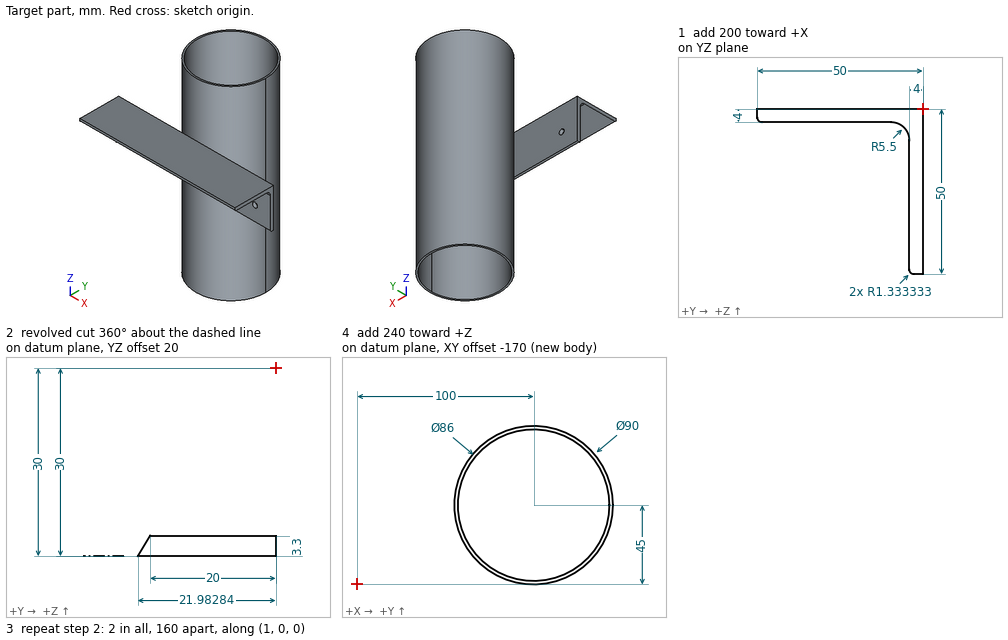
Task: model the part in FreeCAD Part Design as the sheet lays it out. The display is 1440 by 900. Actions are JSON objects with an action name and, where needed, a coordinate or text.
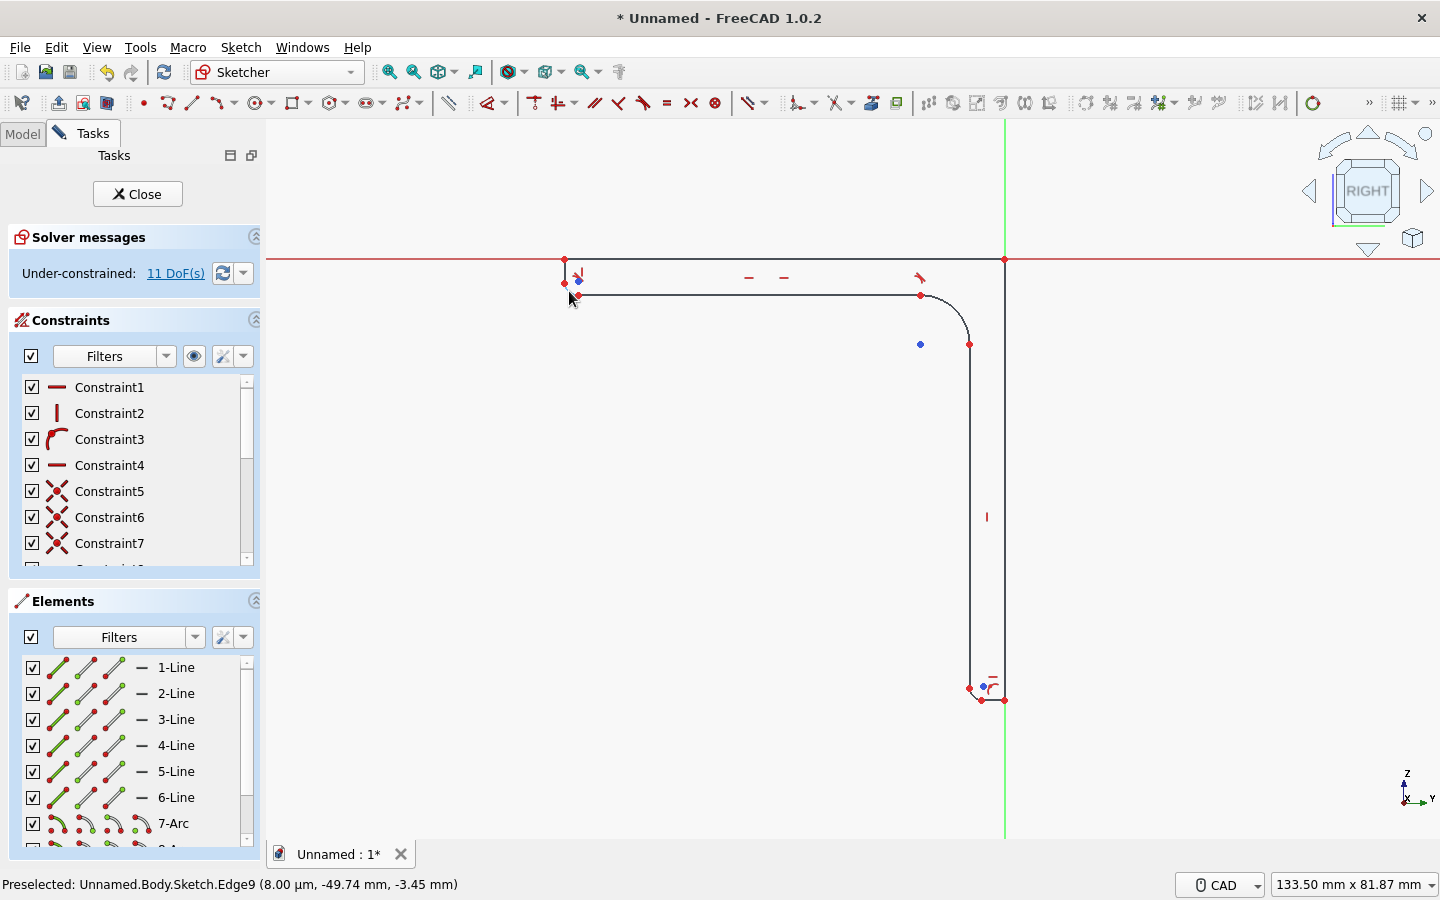
{"action": "left_click", "coordinate": [970, 448]}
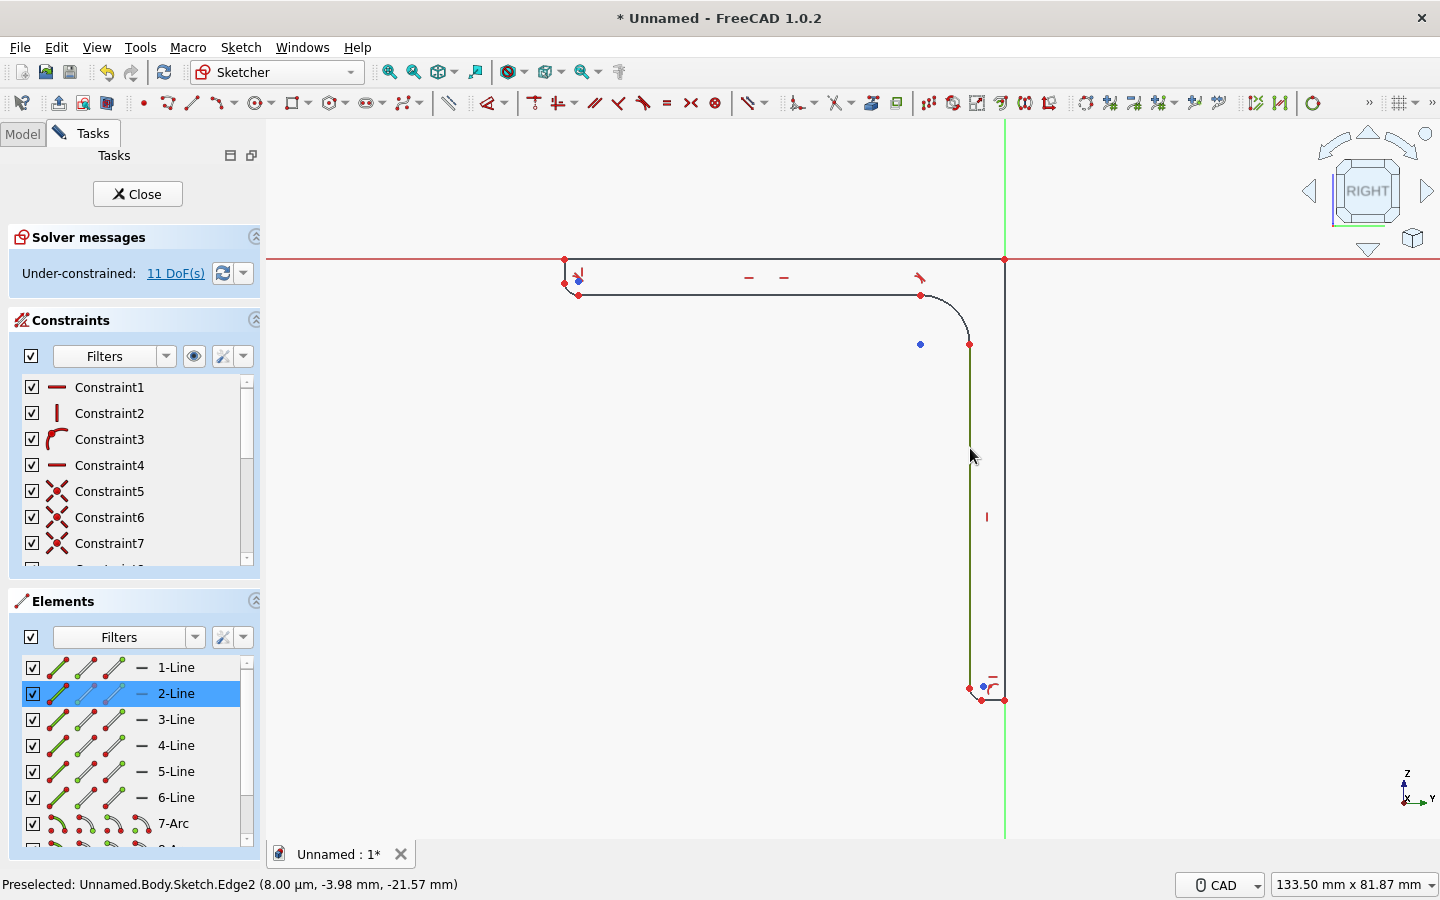
{"action": "left_click", "coordinate": [964, 322]}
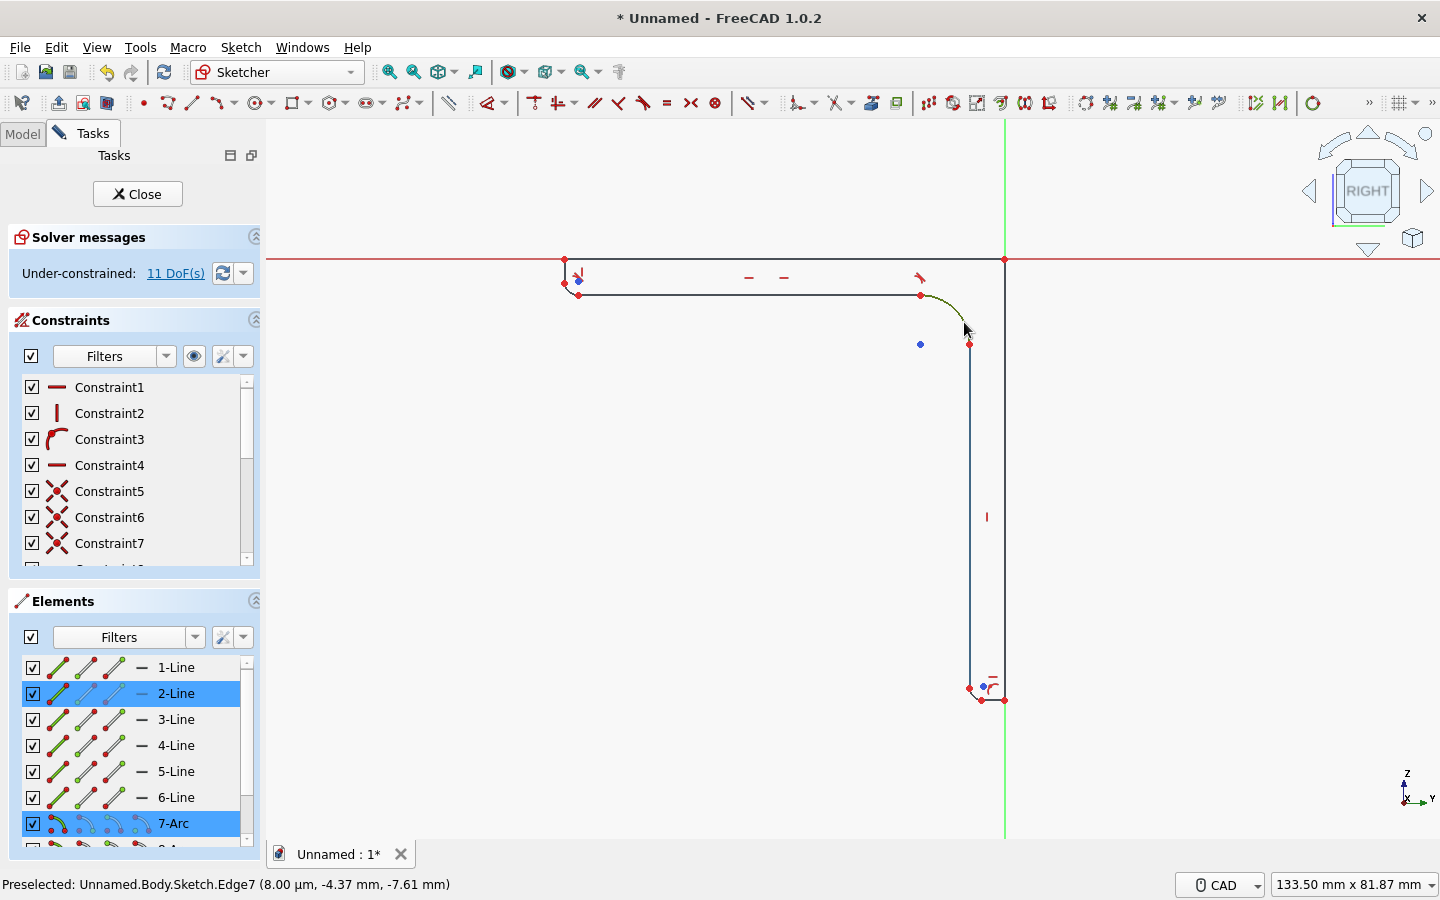
{"action": "left_click", "coordinate": [644, 104]}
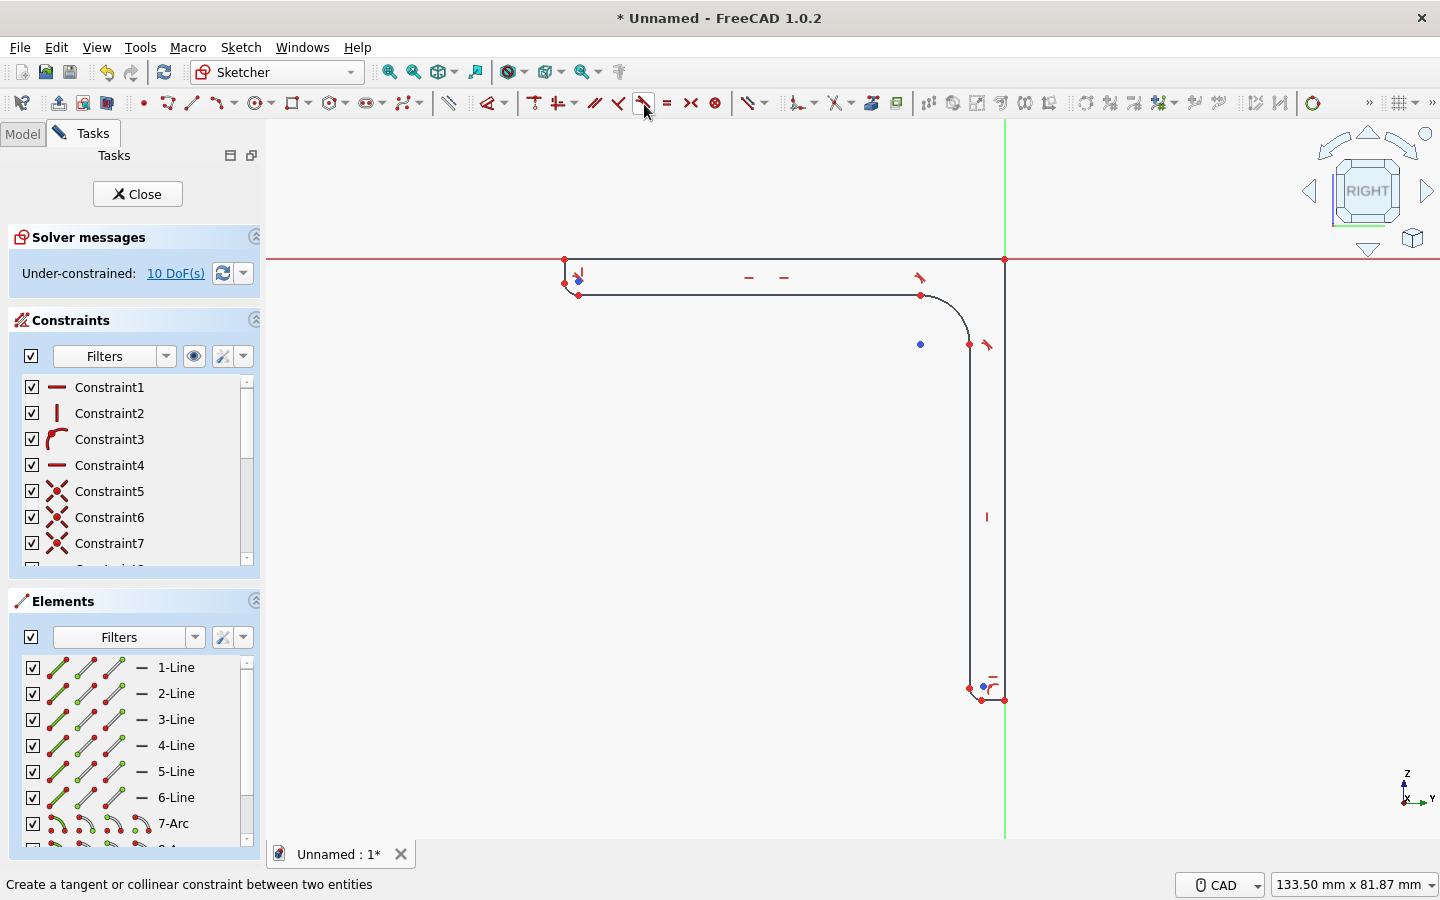
{"action": "left_click", "coordinate": [970, 448]}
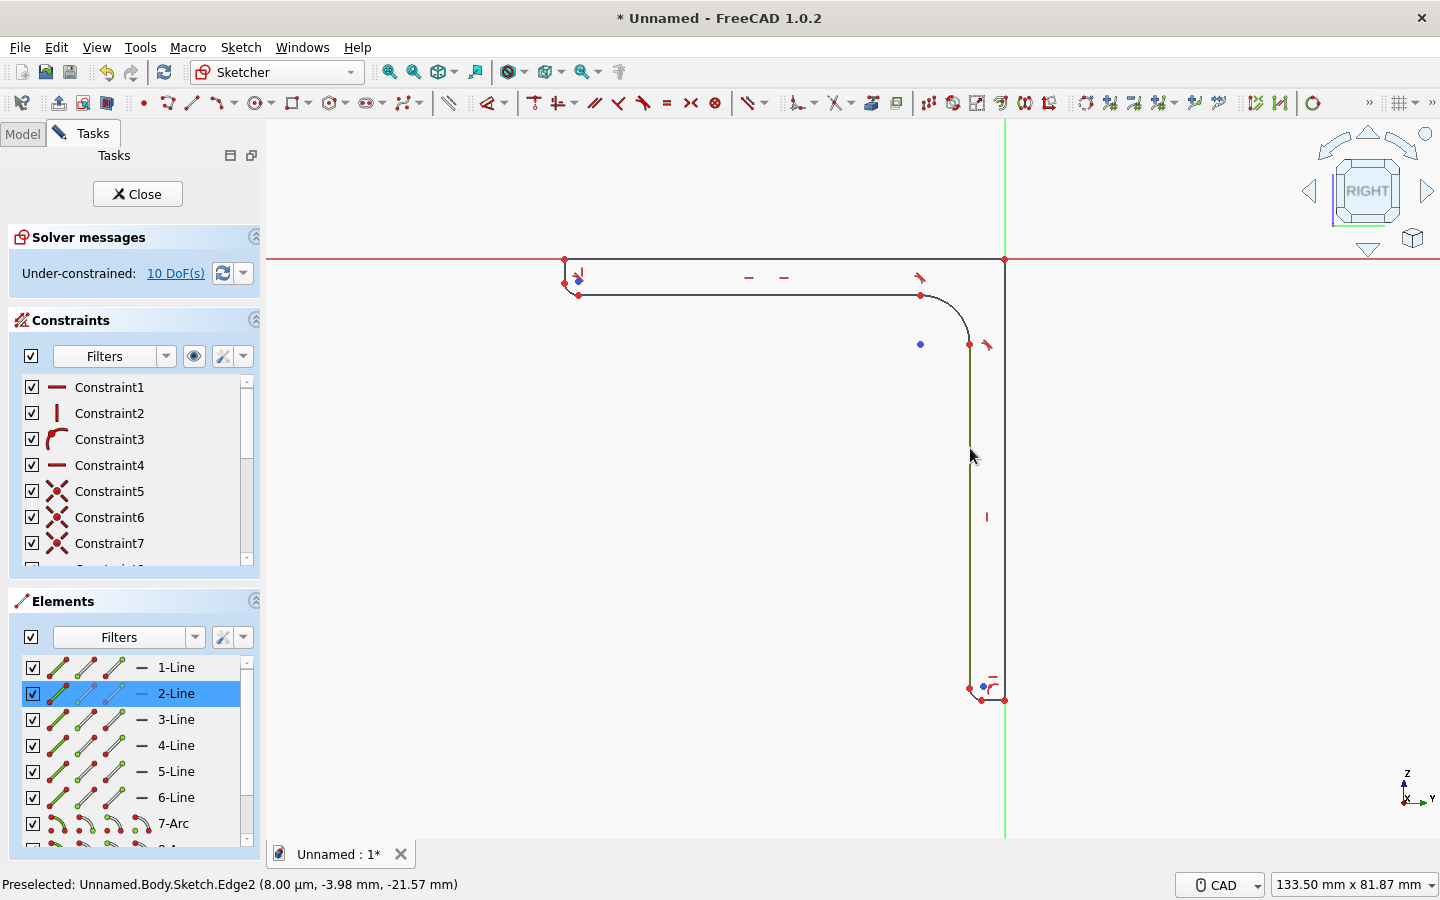
{"action": "scroll", "coordinate": [974, 696], "scroll_direction": "up", "scroll_amount": 3}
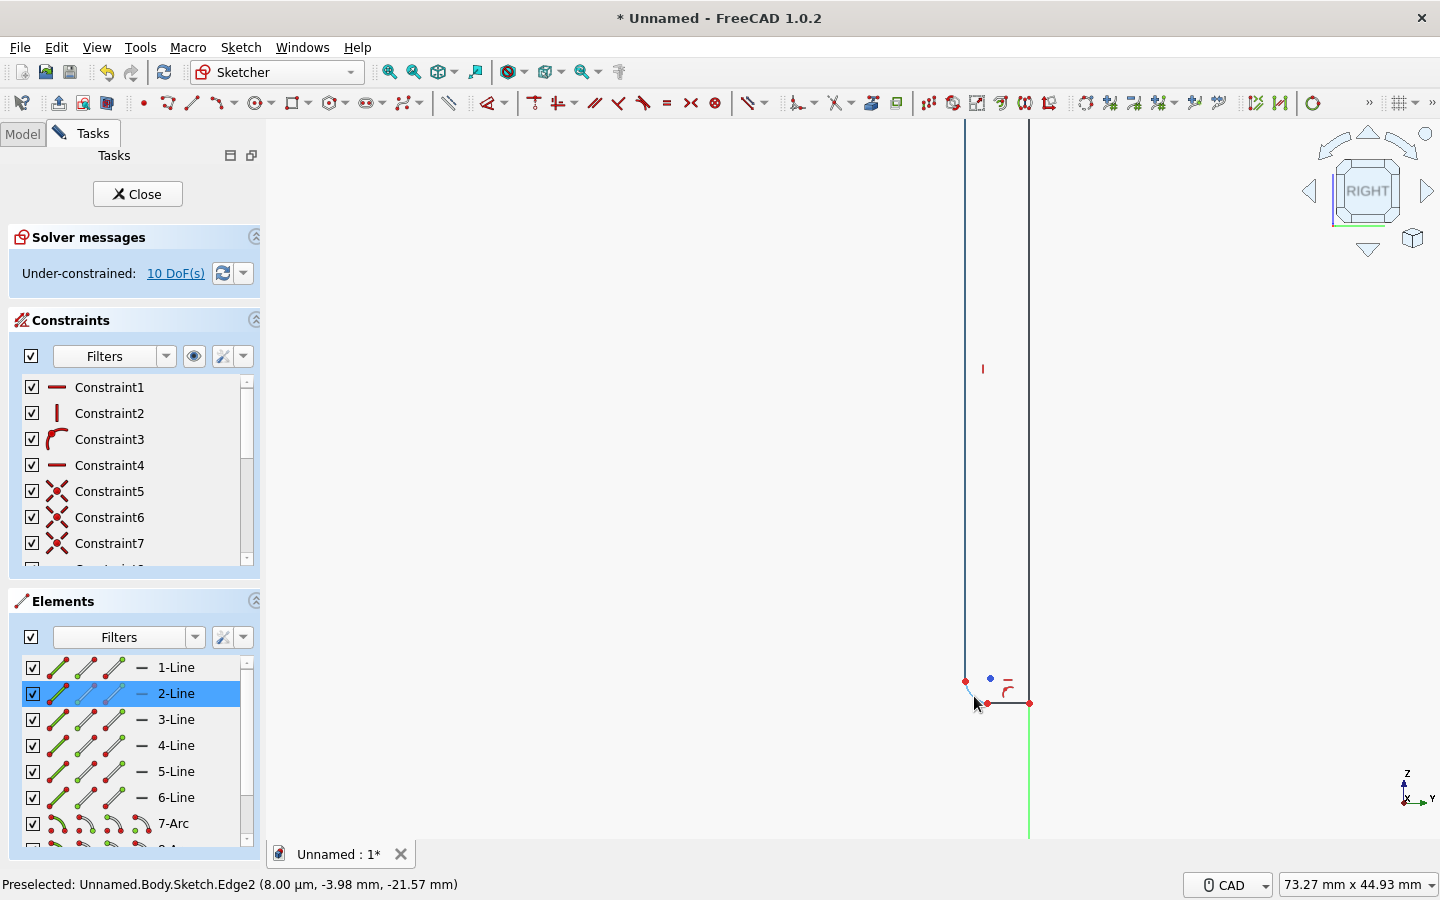
{"action": "left_click", "coordinate": [973, 696]}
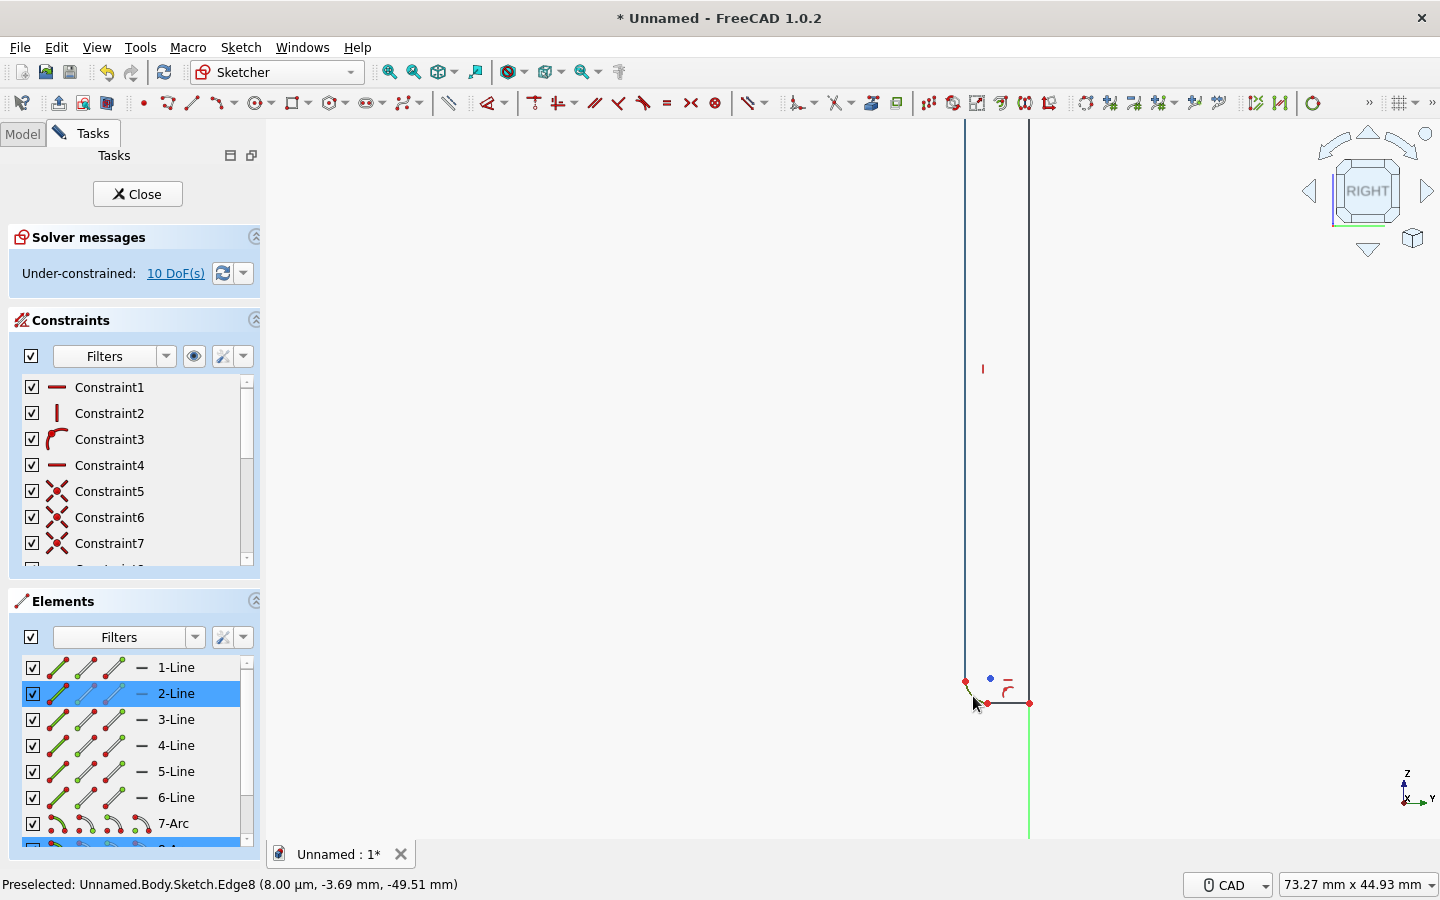
{"action": "left_click", "coordinate": [644, 104]}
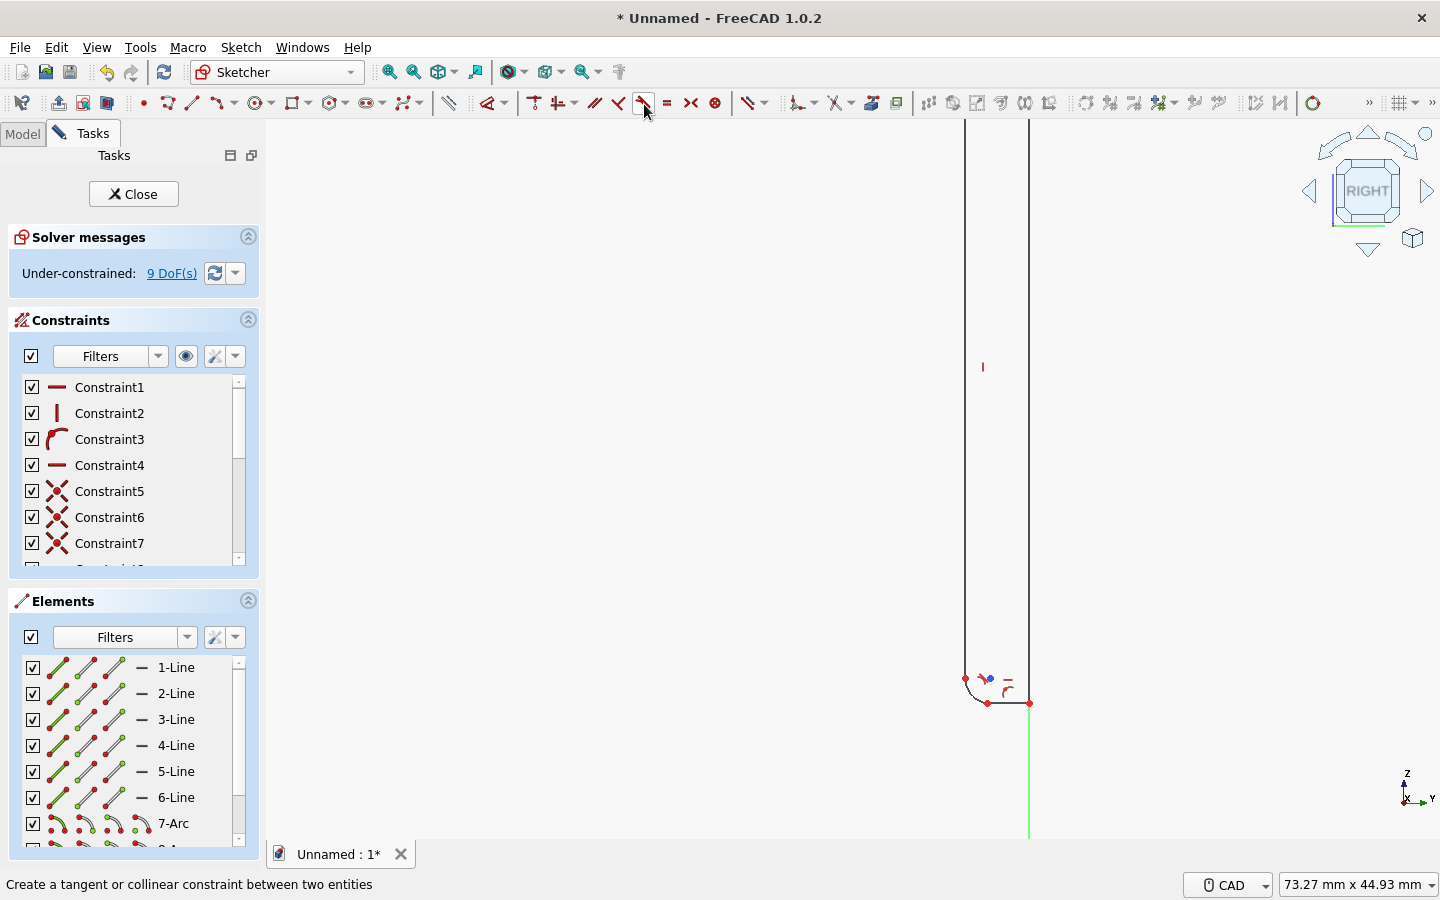
{"action": "left_click", "coordinate": [1000, 703]}